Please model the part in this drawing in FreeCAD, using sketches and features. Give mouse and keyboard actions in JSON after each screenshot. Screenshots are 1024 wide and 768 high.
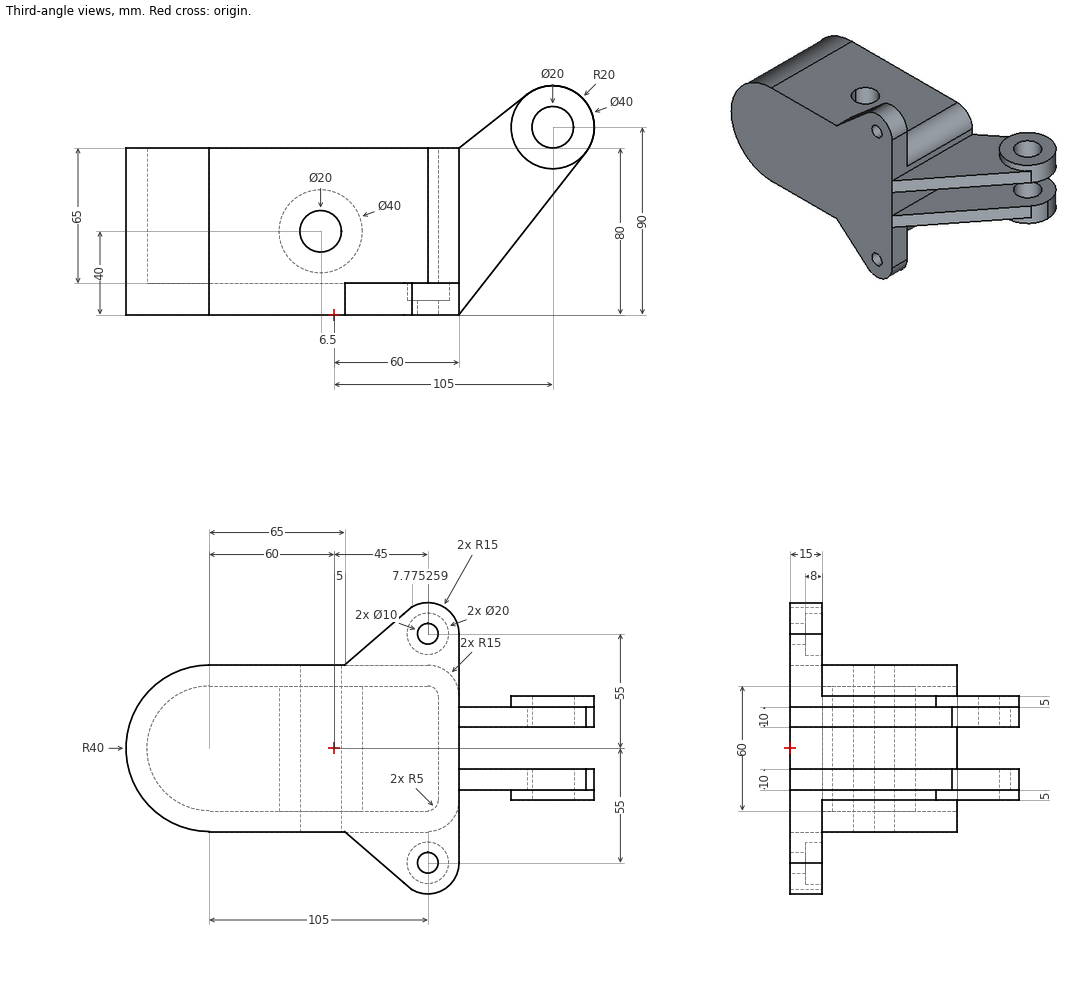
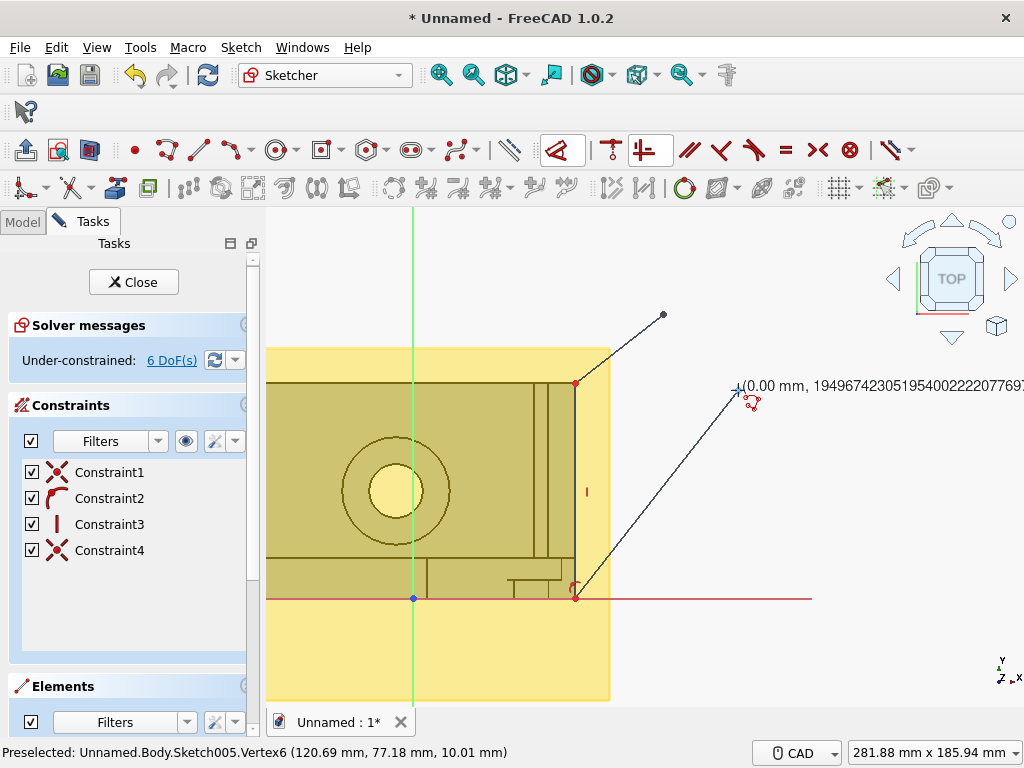
{"action": "left_click", "coordinate": [232, 150]}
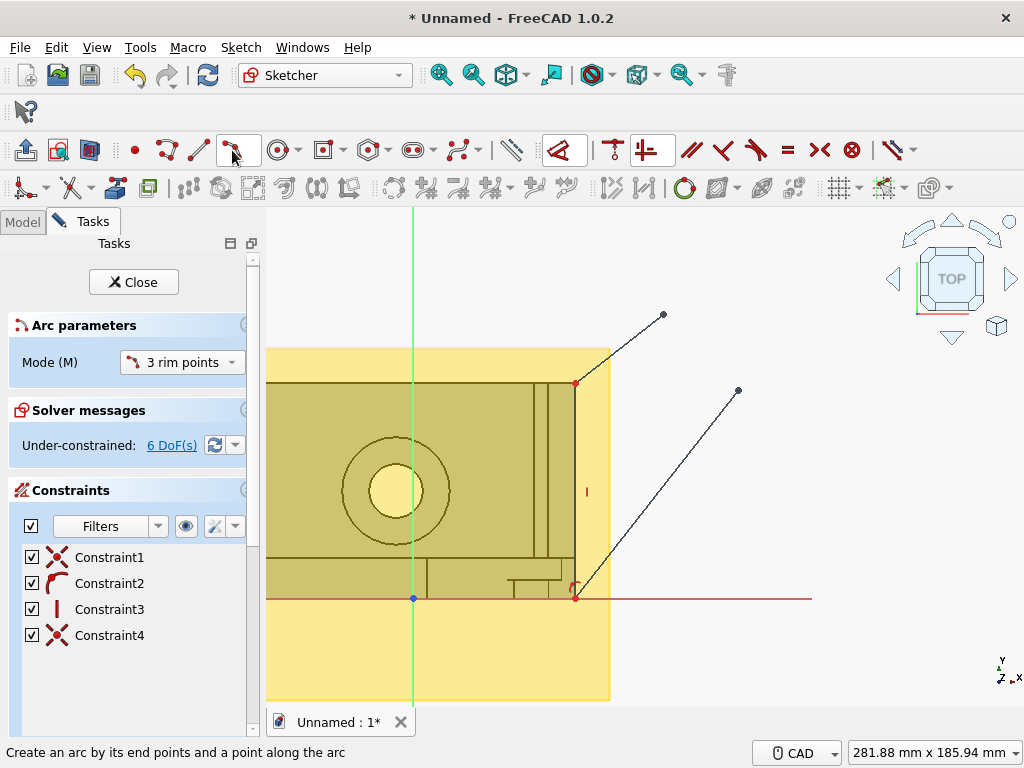
{"action": "left_click", "coordinate": [738, 391]}
{"action": "left_click", "coordinate": [663, 315]}
{"action": "left_click", "coordinate": [734, 318]}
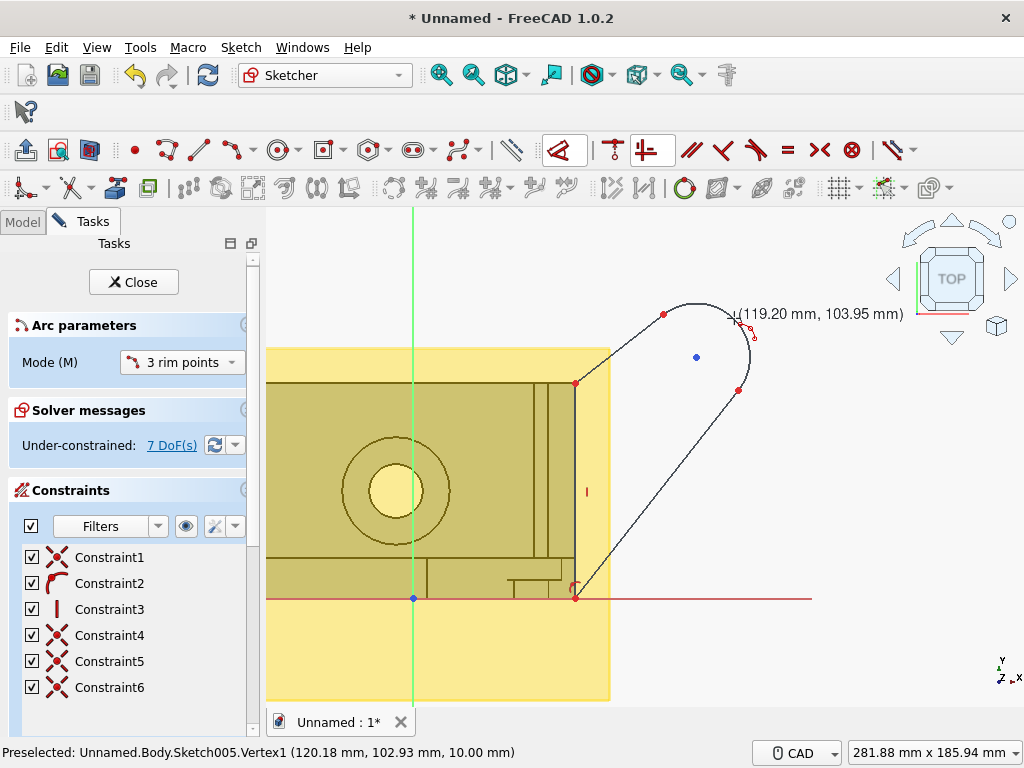
{"action": "left_click", "coordinate": [278, 150]}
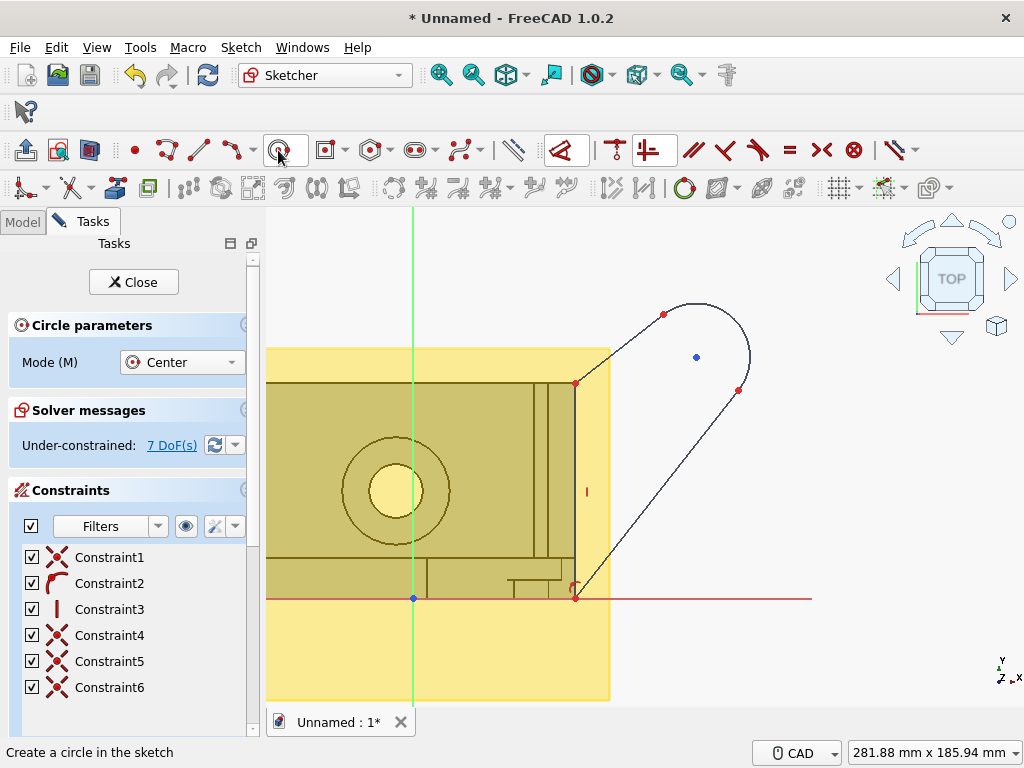
{"action": "left_click", "coordinate": [696, 357]}
{"action": "left_click", "coordinate": [715, 338]}
{"action": "key", "text": "Escape"}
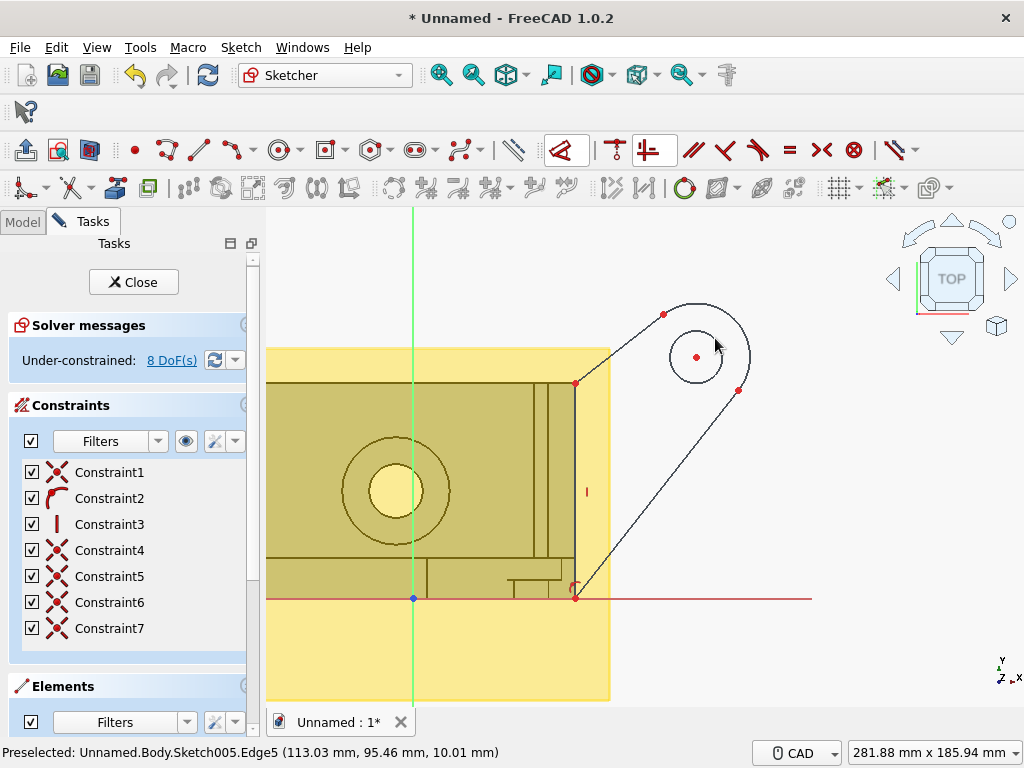
{"action": "left_click", "coordinate": [637, 336]}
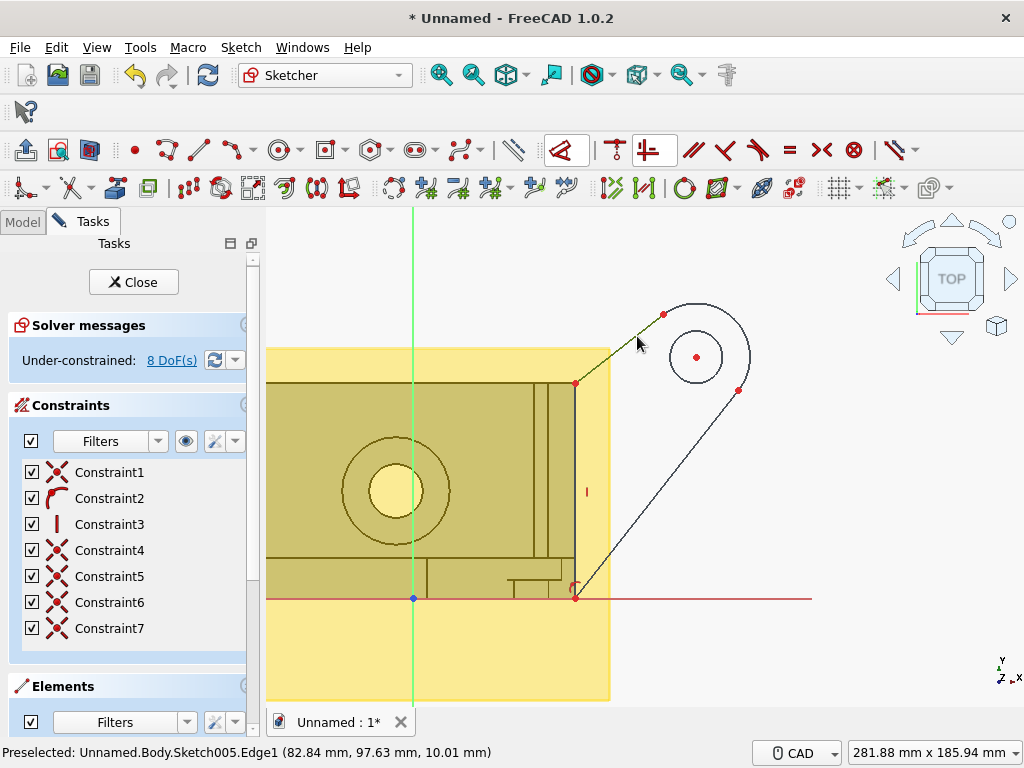
{"action": "left_click", "coordinate": [749, 347]}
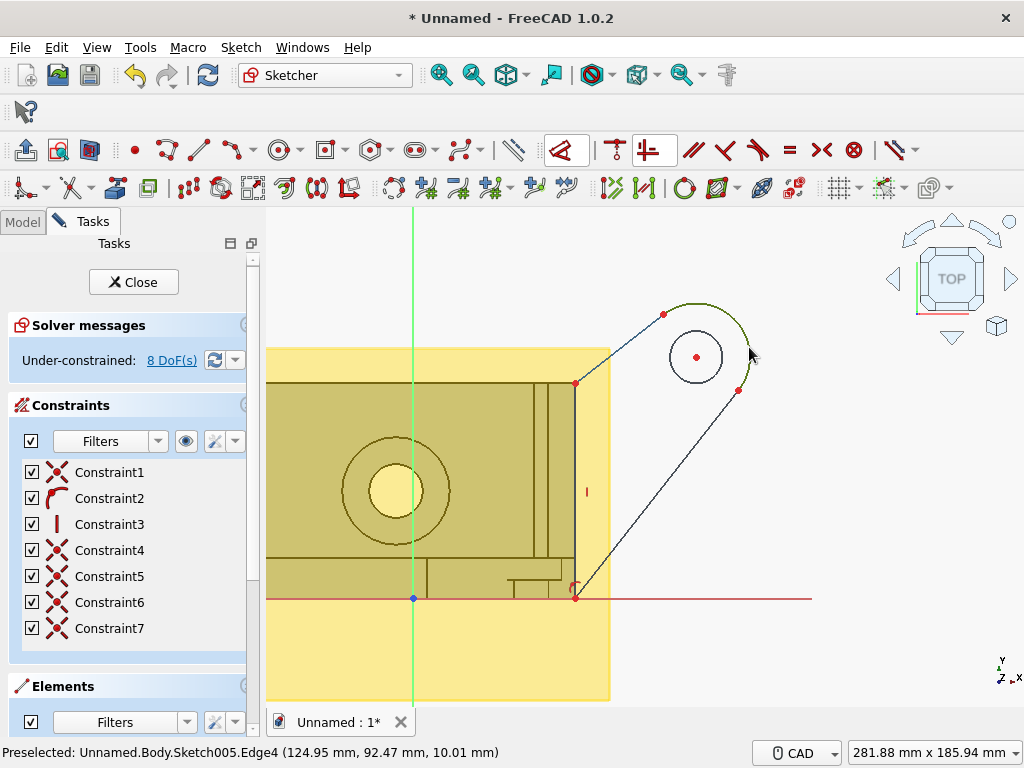
{"action": "left_click", "coordinate": [758, 150]}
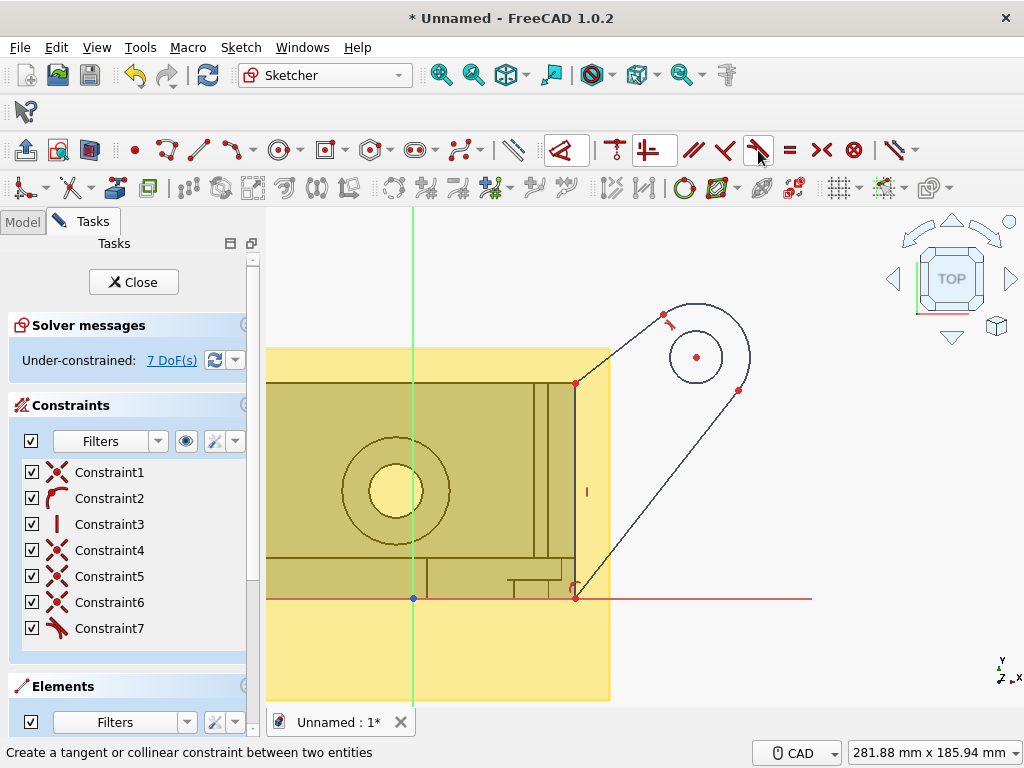
{"action": "left_click", "coordinate": [624, 536]}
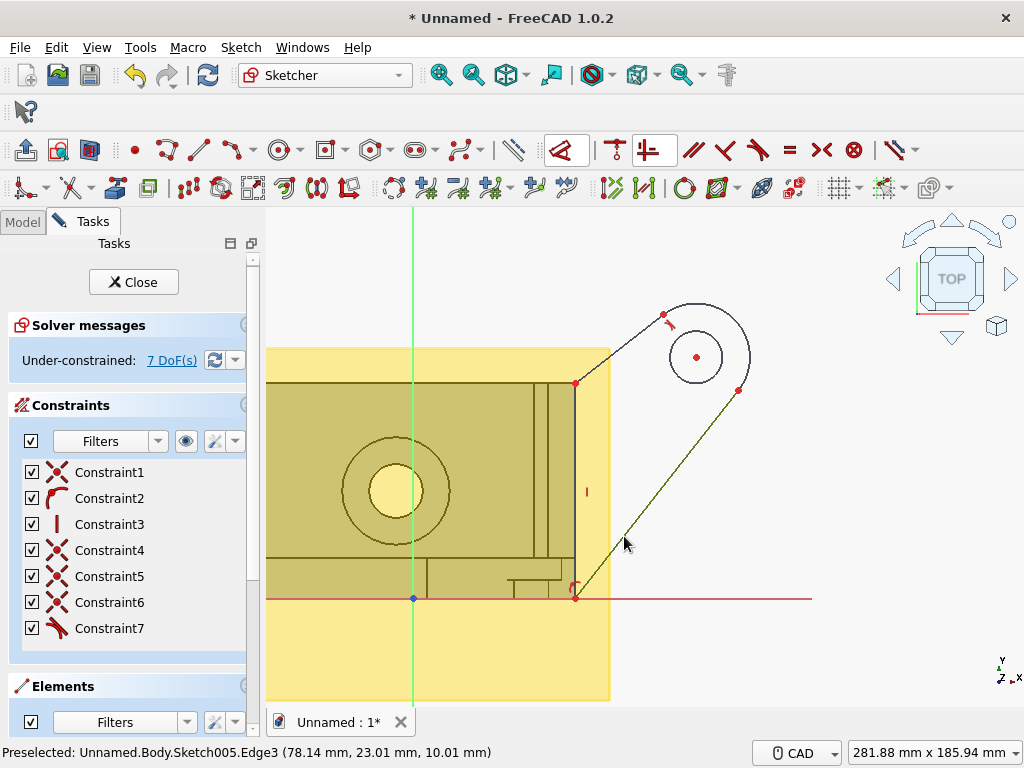
{"action": "left_click", "coordinate": [749, 347]}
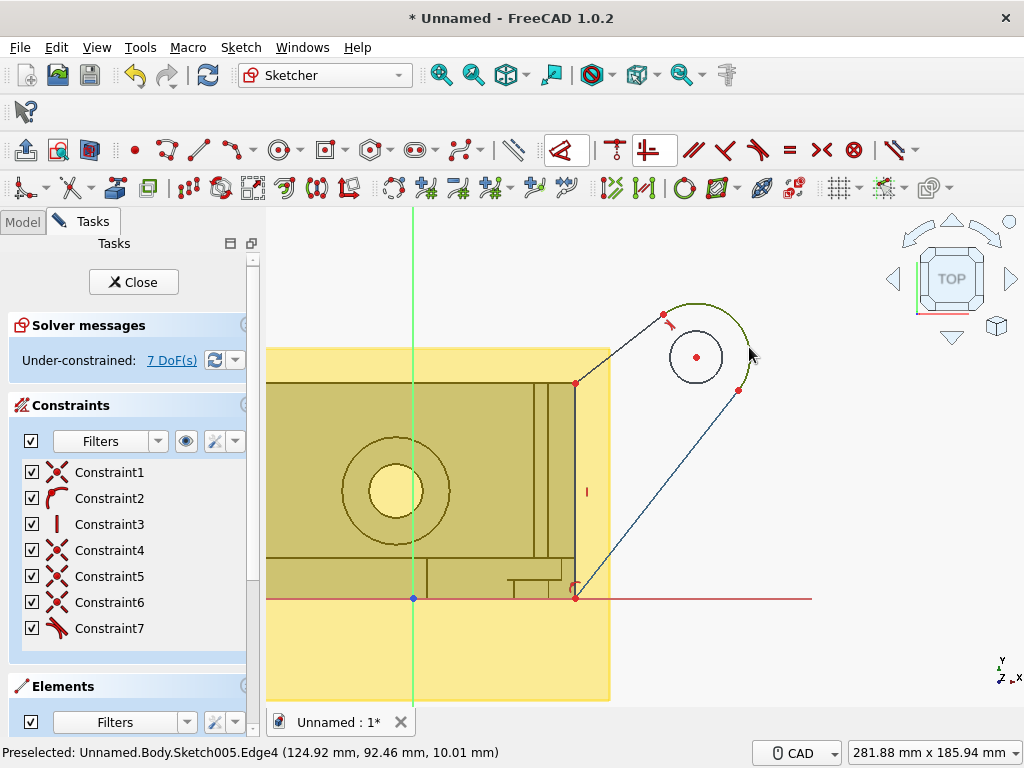
{"action": "left_click", "coordinate": [758, 150]}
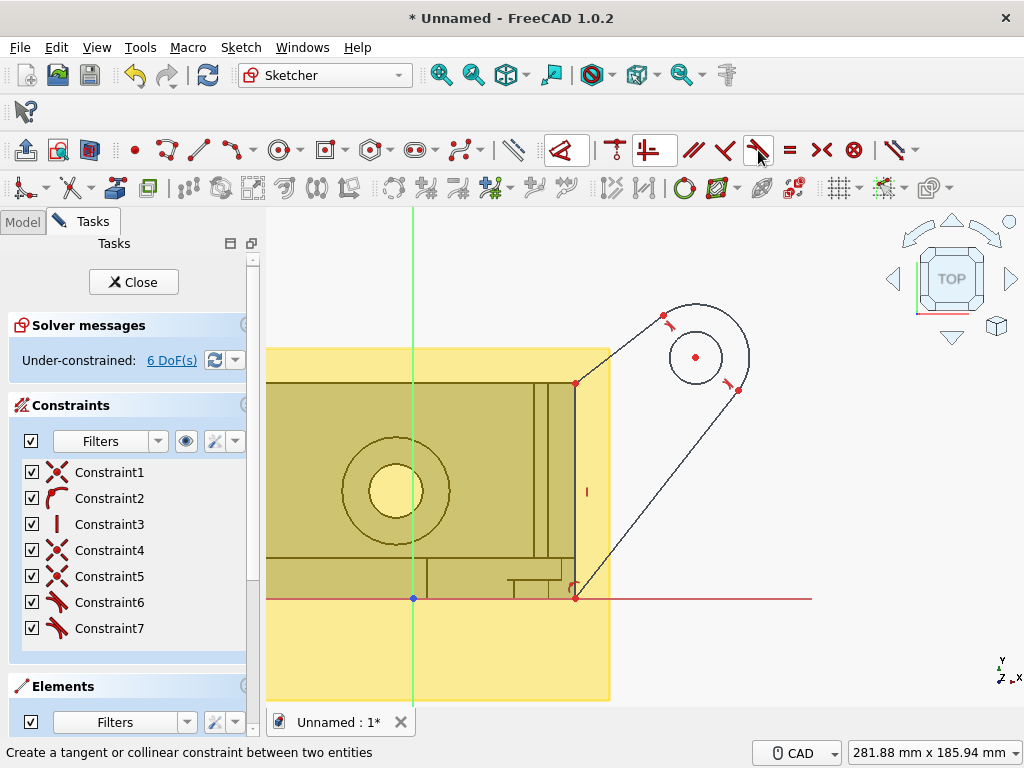
{"action": "left_click", "coordinate": [748, 347]}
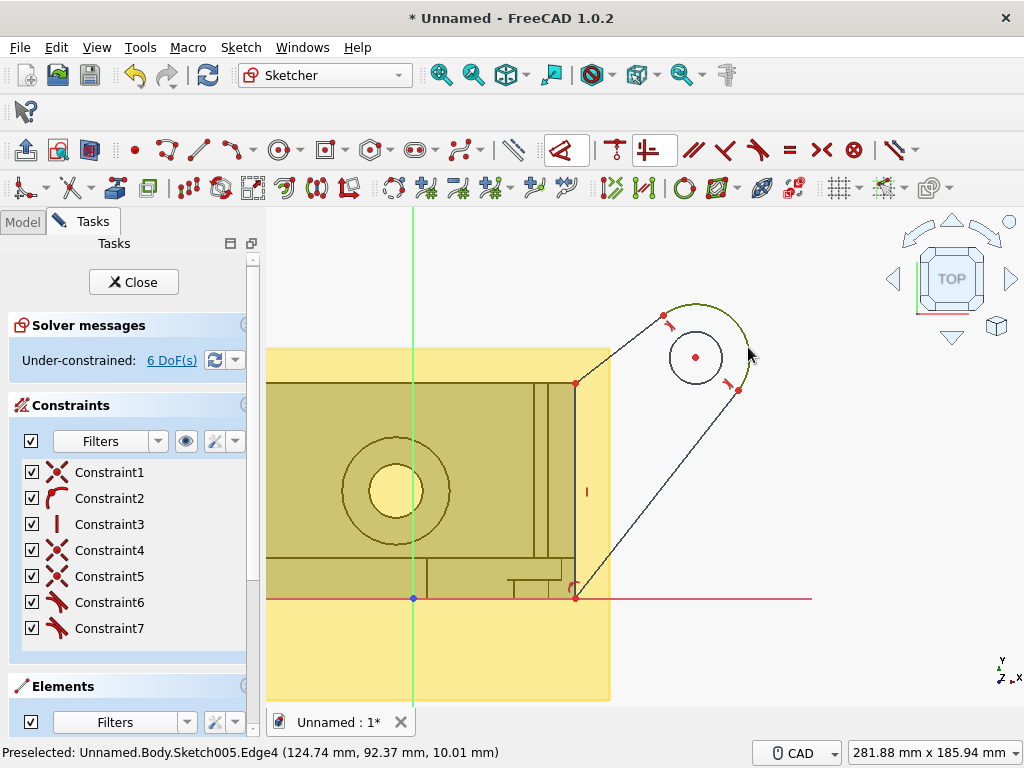
{"action": "key", "text": "k r"}